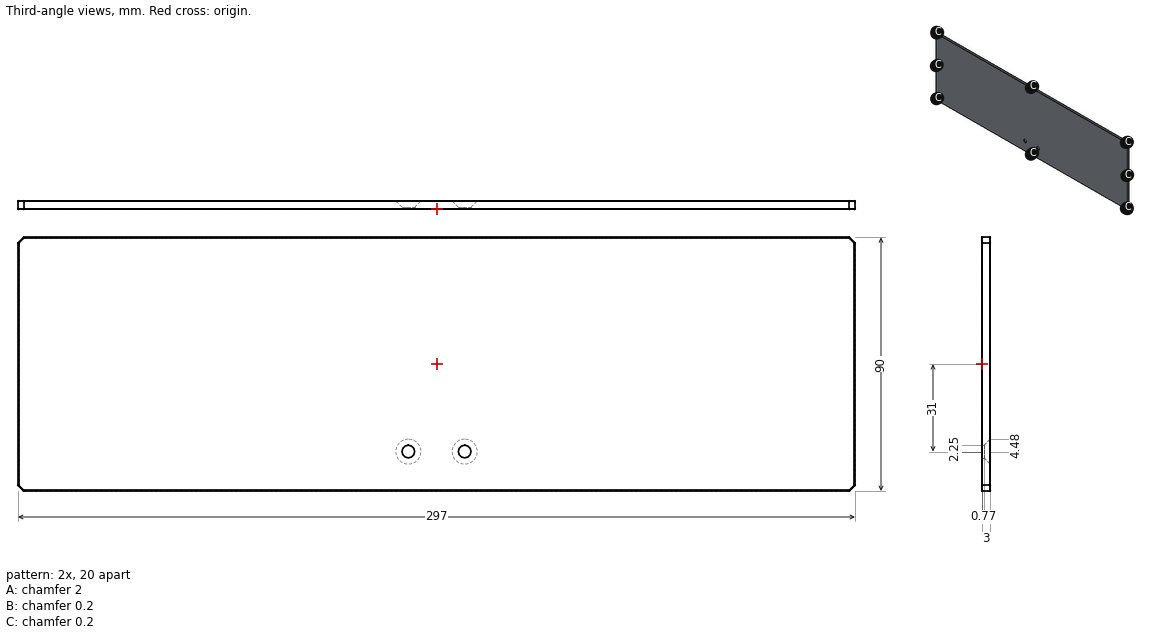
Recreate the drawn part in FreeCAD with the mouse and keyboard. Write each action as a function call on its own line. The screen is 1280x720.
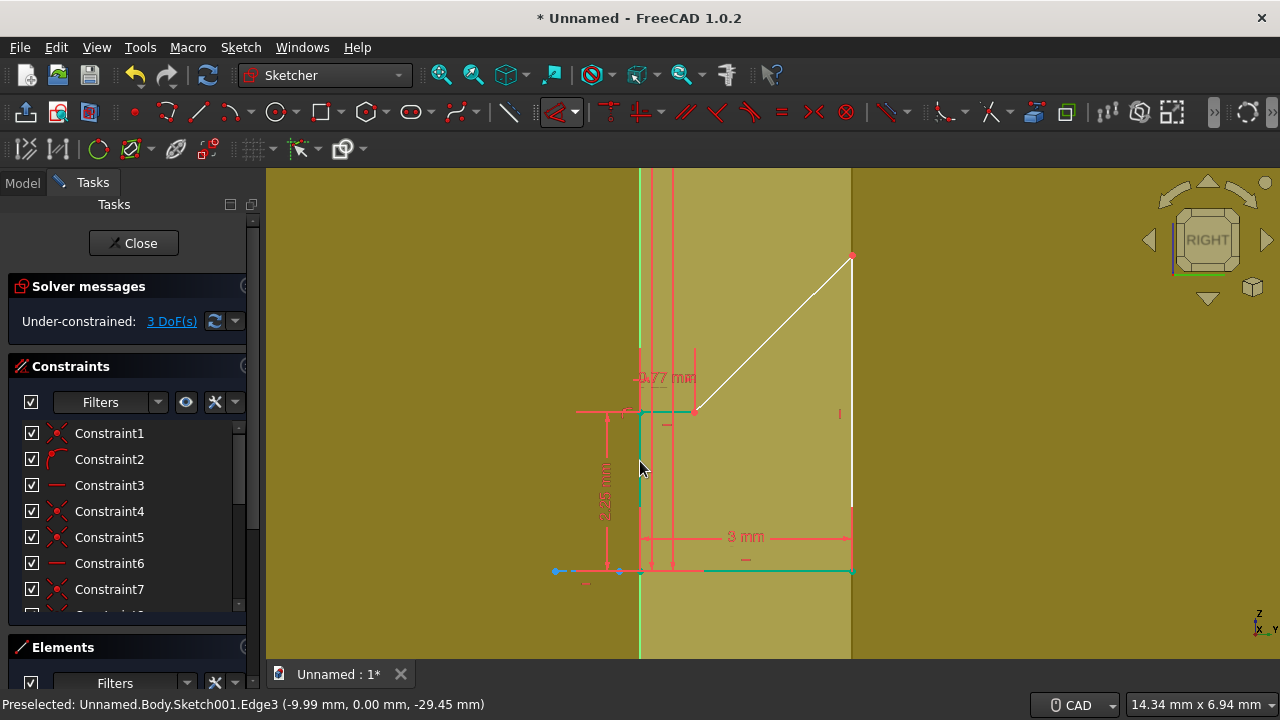
click(852, 477)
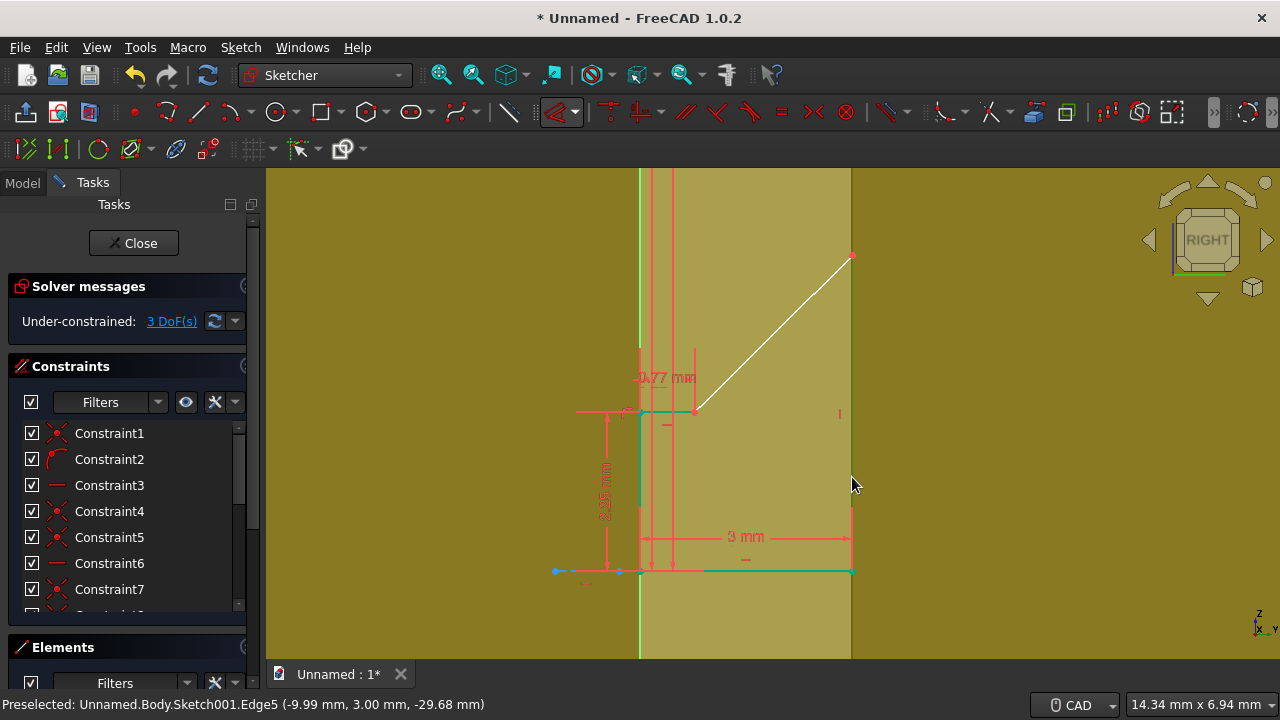
click(578, 112)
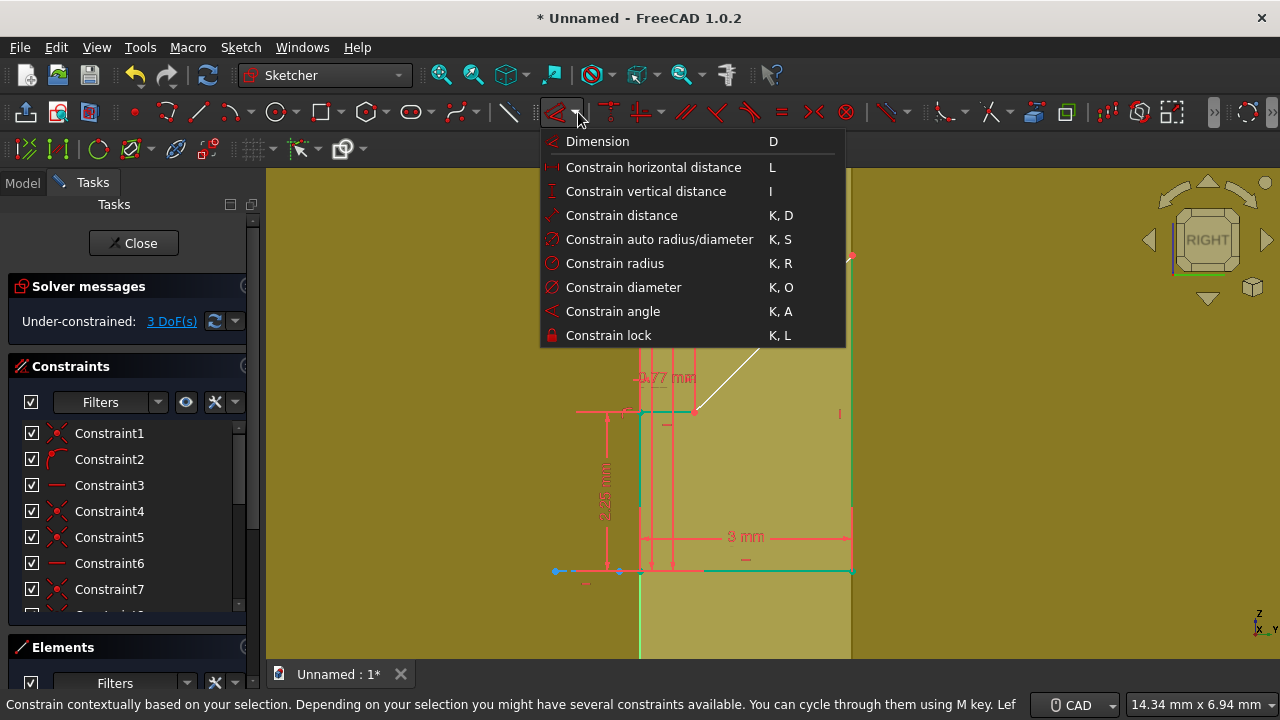
click(693, 191)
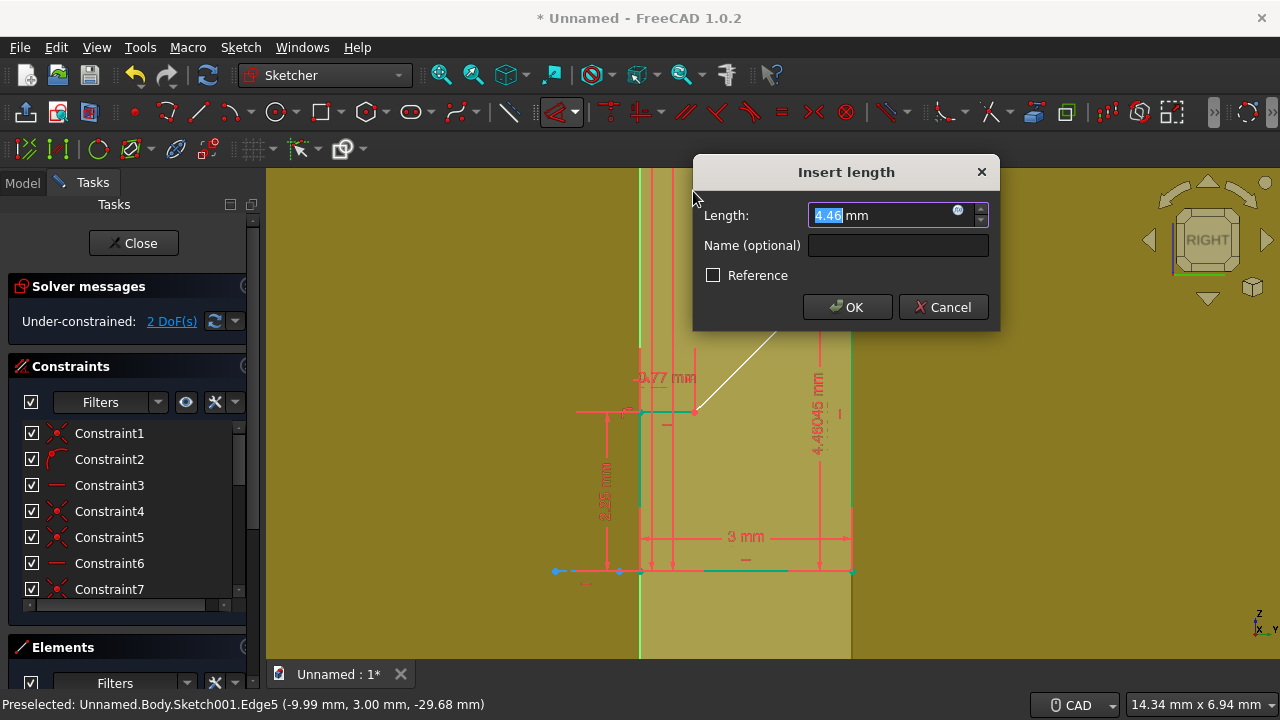
text(4.48)
key(Return)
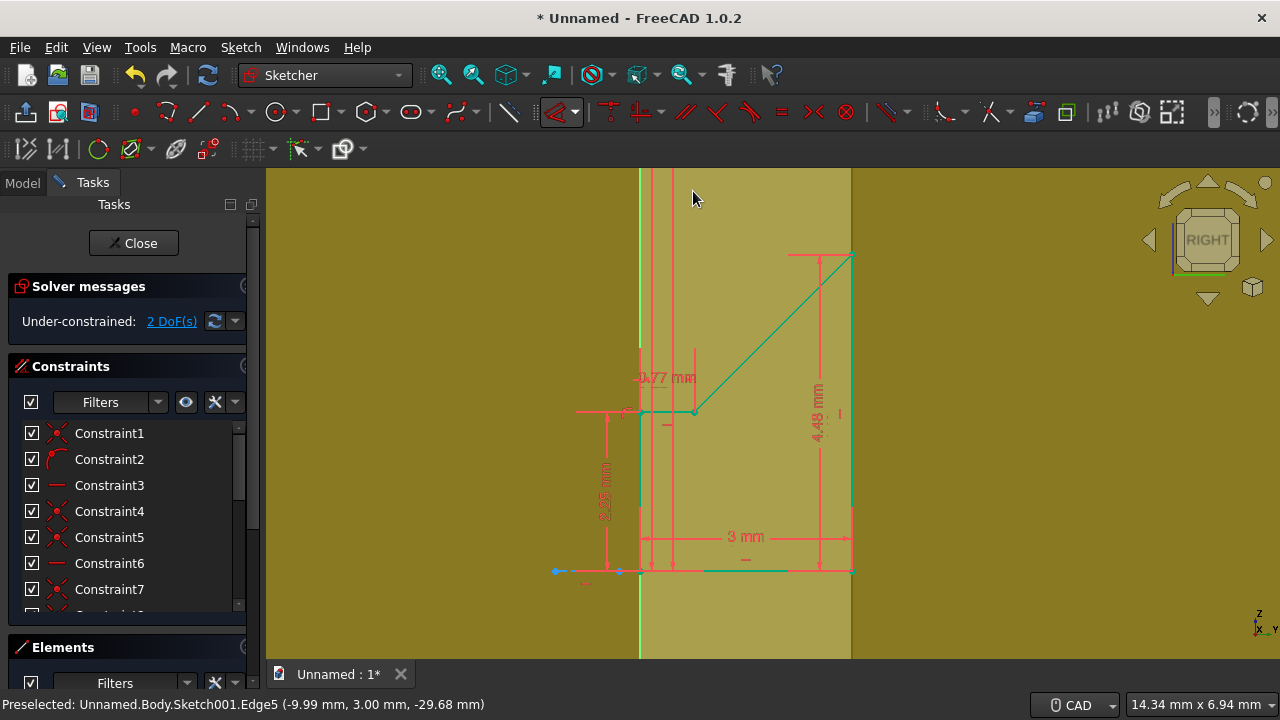
click(134, 243)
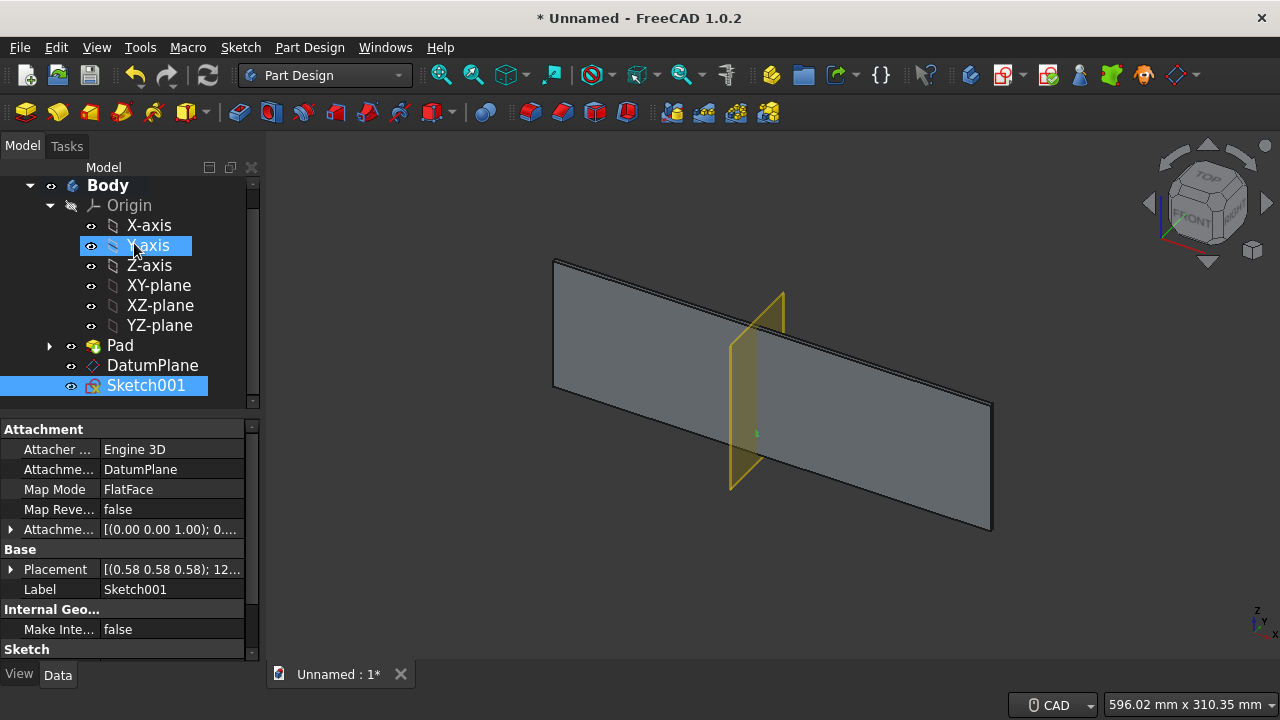
click(304, 112)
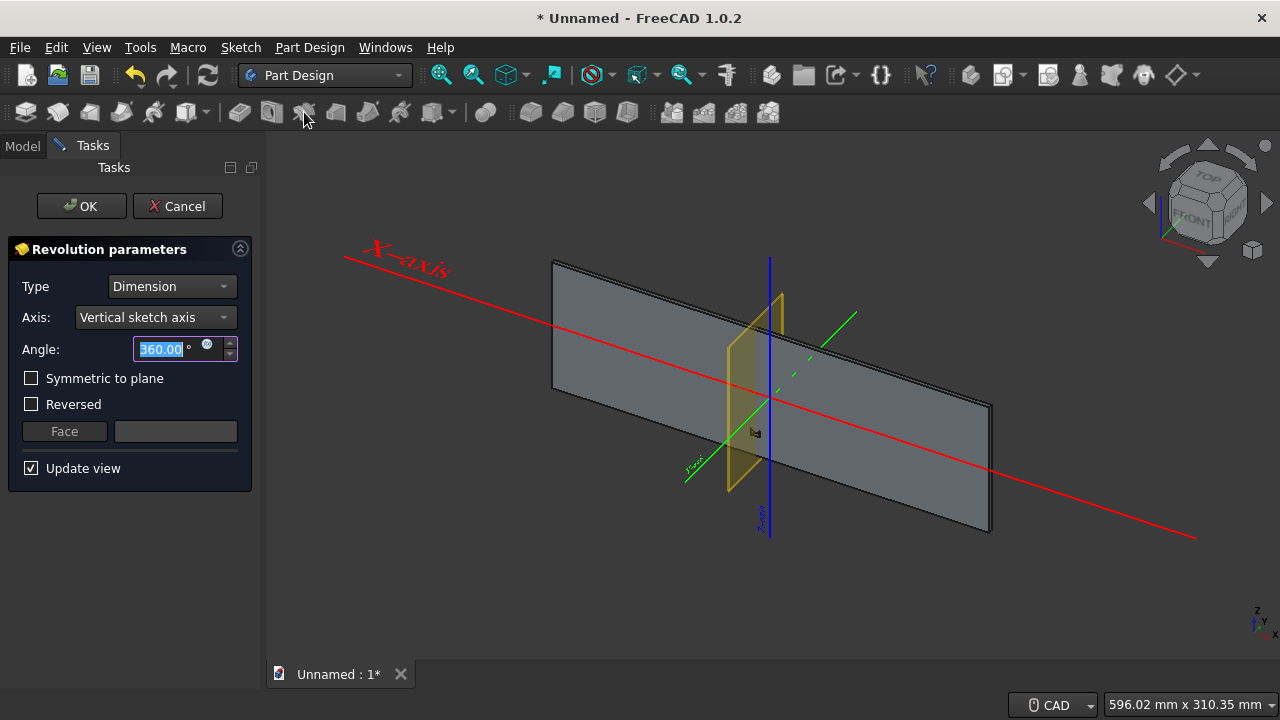
click(156, 318)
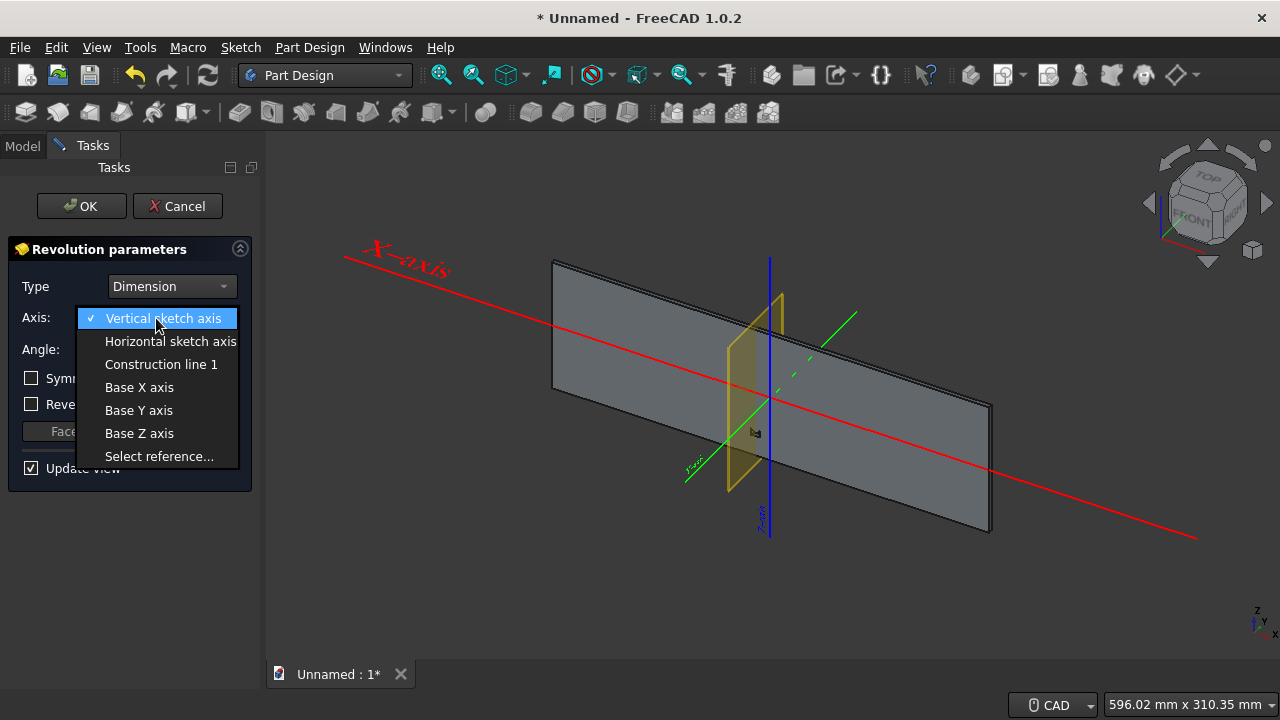
click(156, 364)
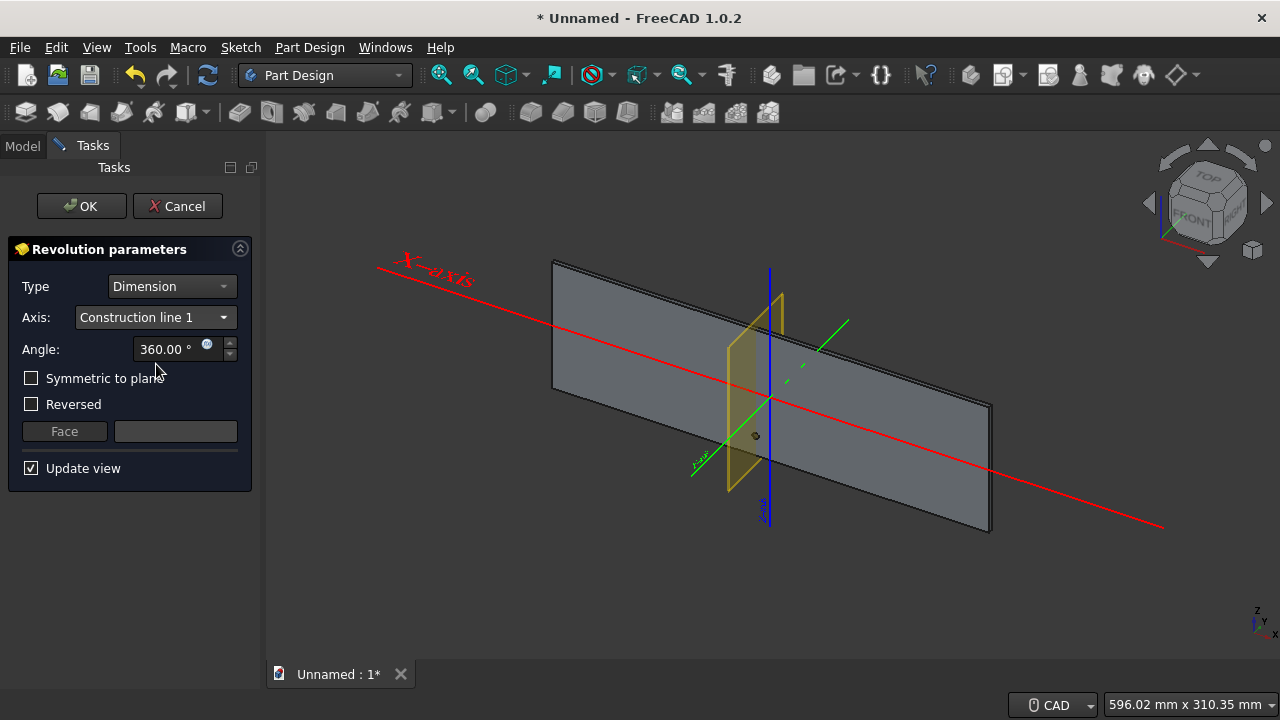
click(82, 206)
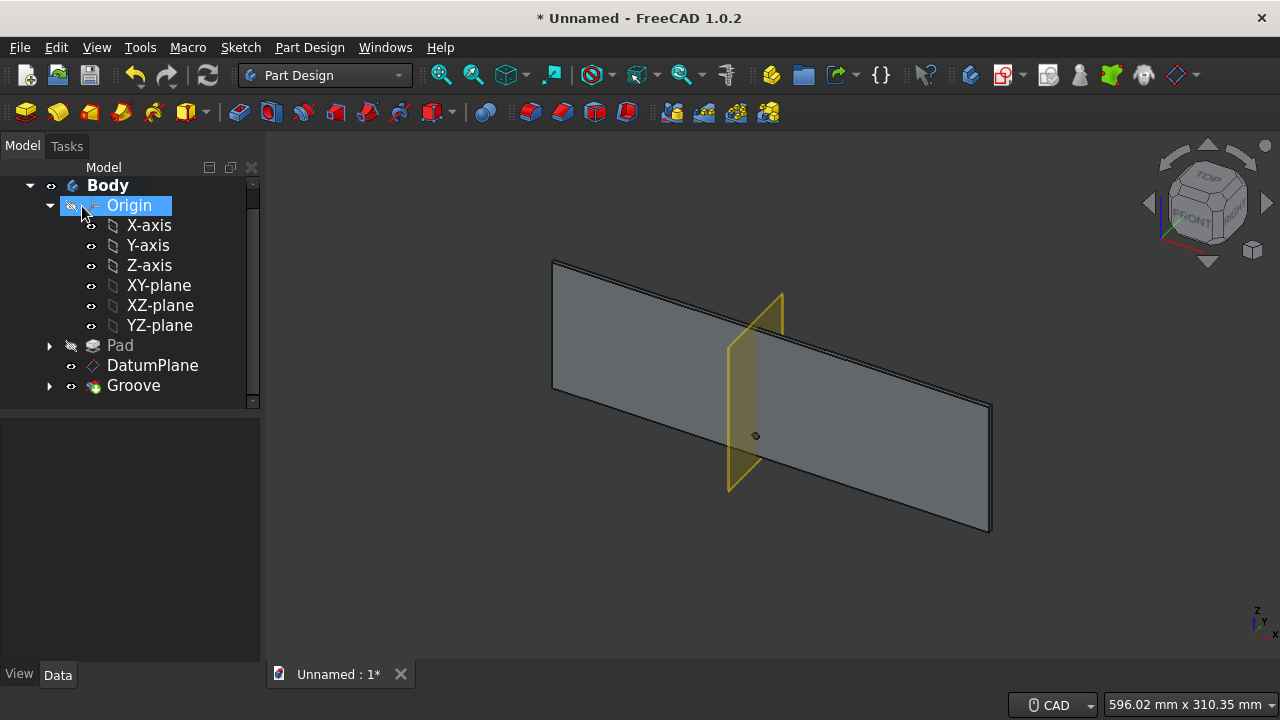
click(116, 366)
key(space)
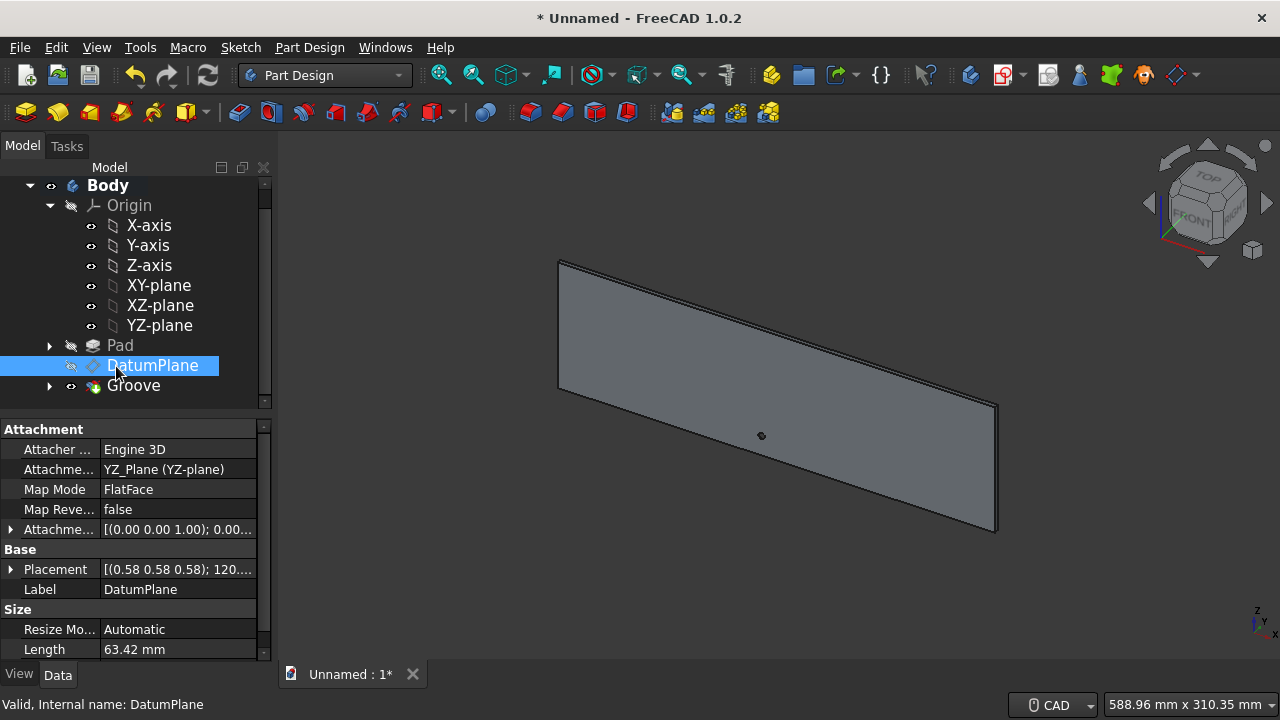
click(116, 386)